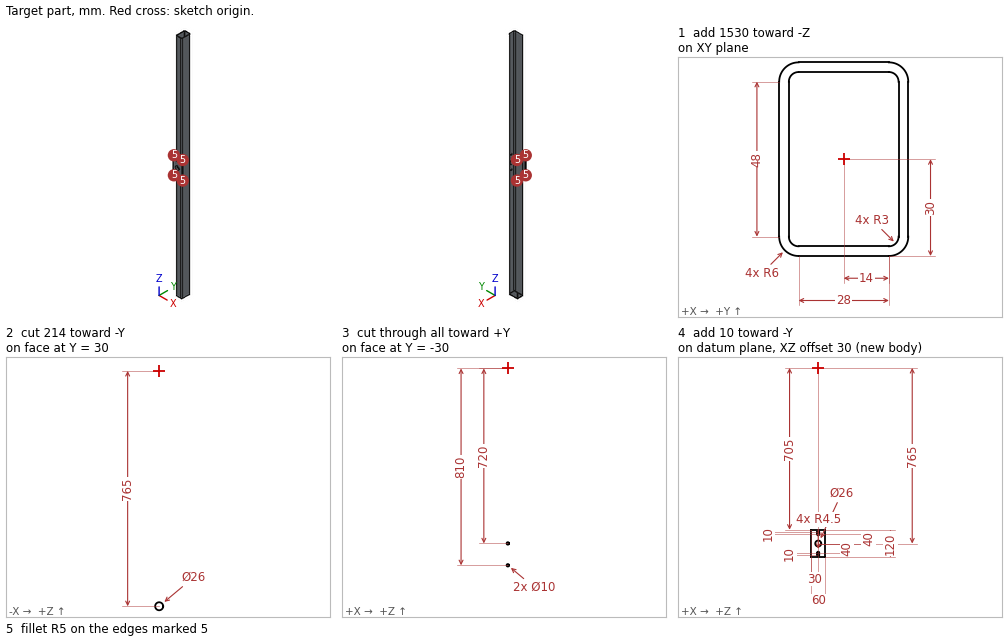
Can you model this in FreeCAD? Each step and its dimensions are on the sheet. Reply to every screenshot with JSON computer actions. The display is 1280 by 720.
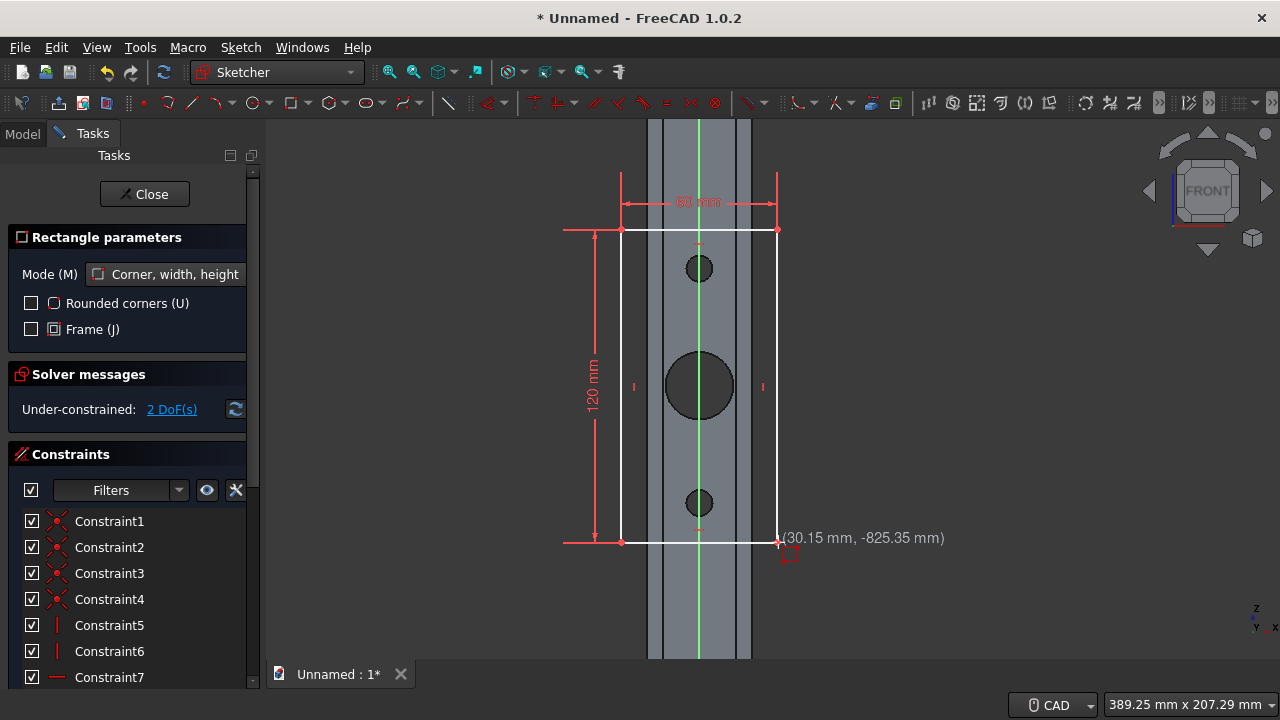
{"action": "left_click", "coordinate": [366, 104]}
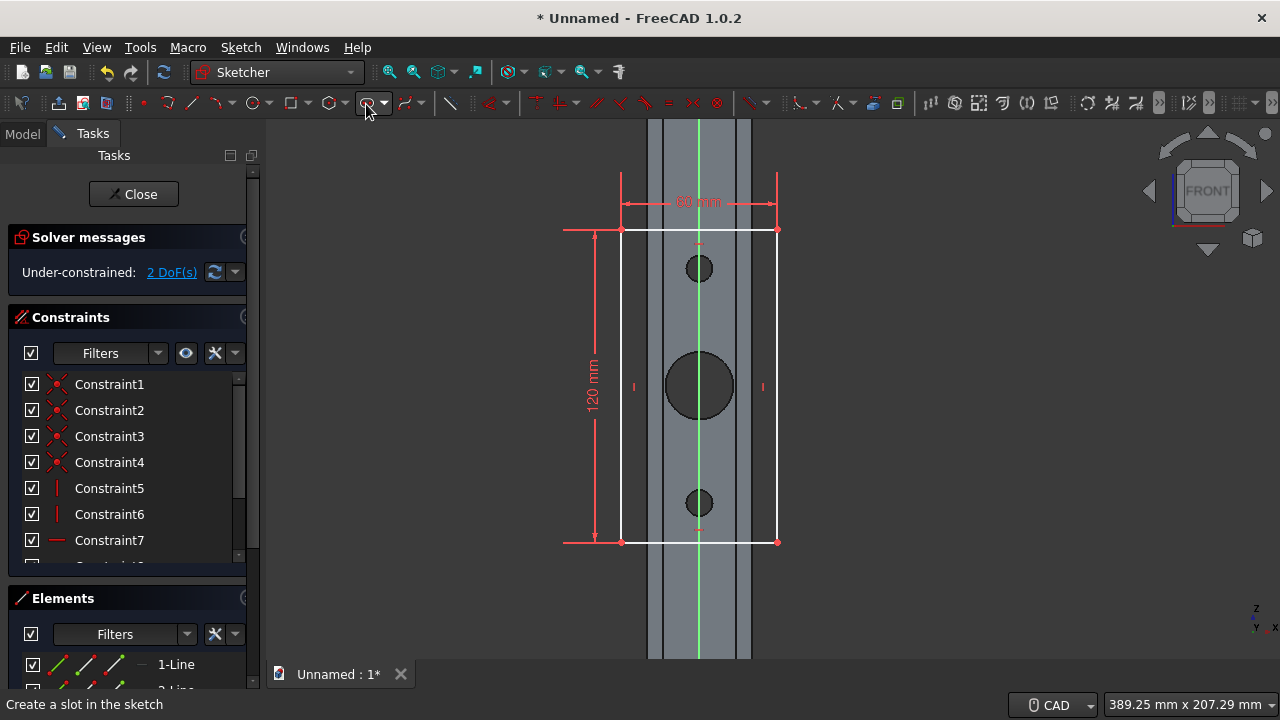
{"action": "scroll", "coordinate": [699, 516], "scroll_direction": "up", "scroll_amount": 4}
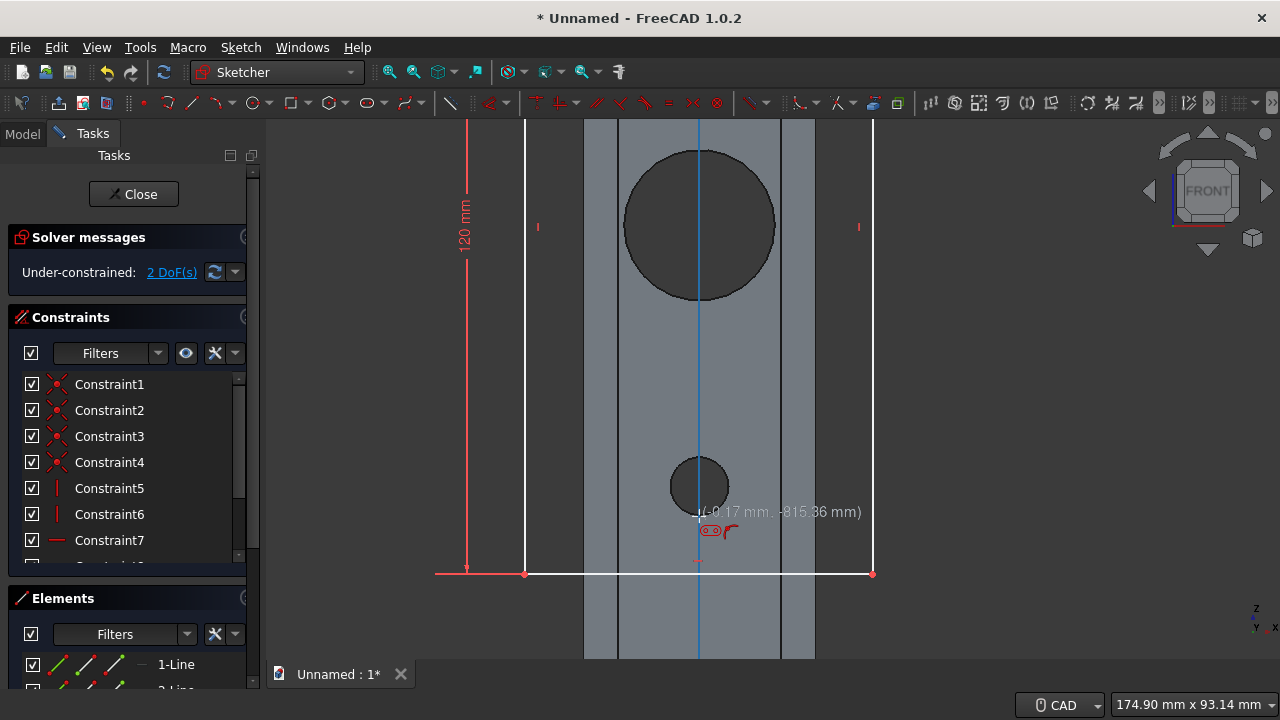
{"action": "left_click", "coordinate": [699, 515]}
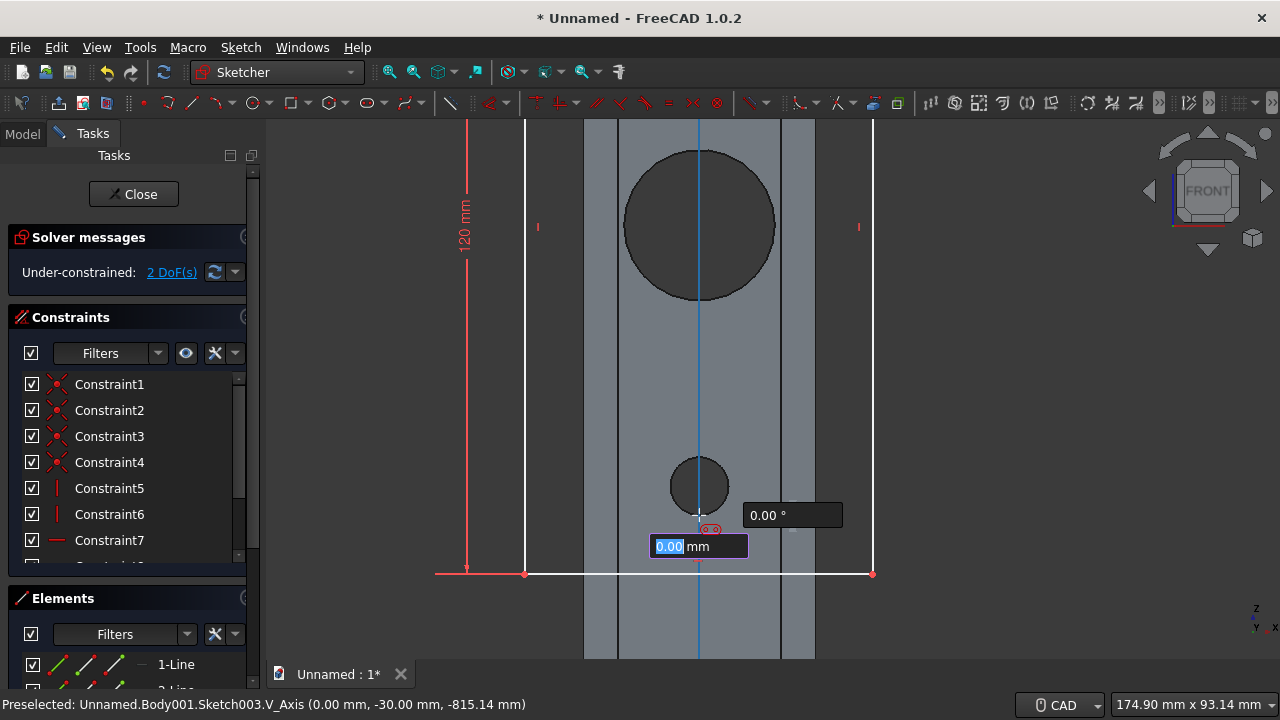
{"action": "left_click", "coordinate": [708, 457]}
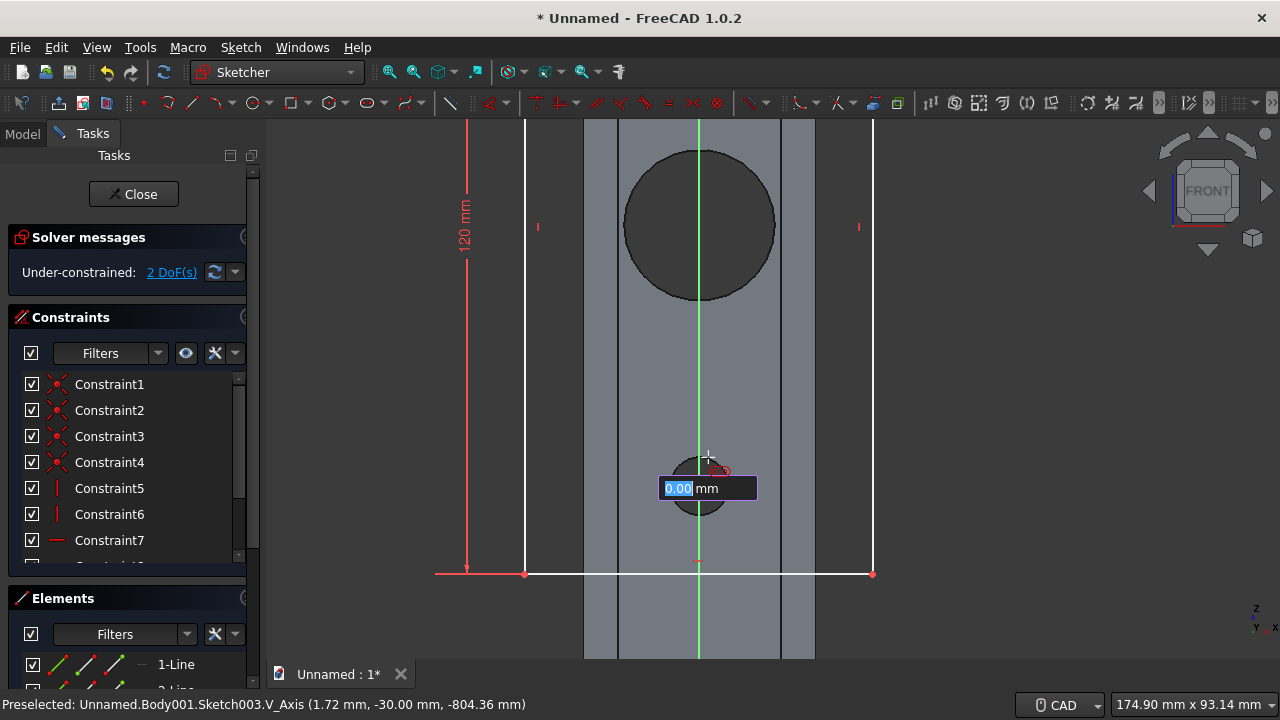
{"action": "left_click", "coordinate": [726, 486]}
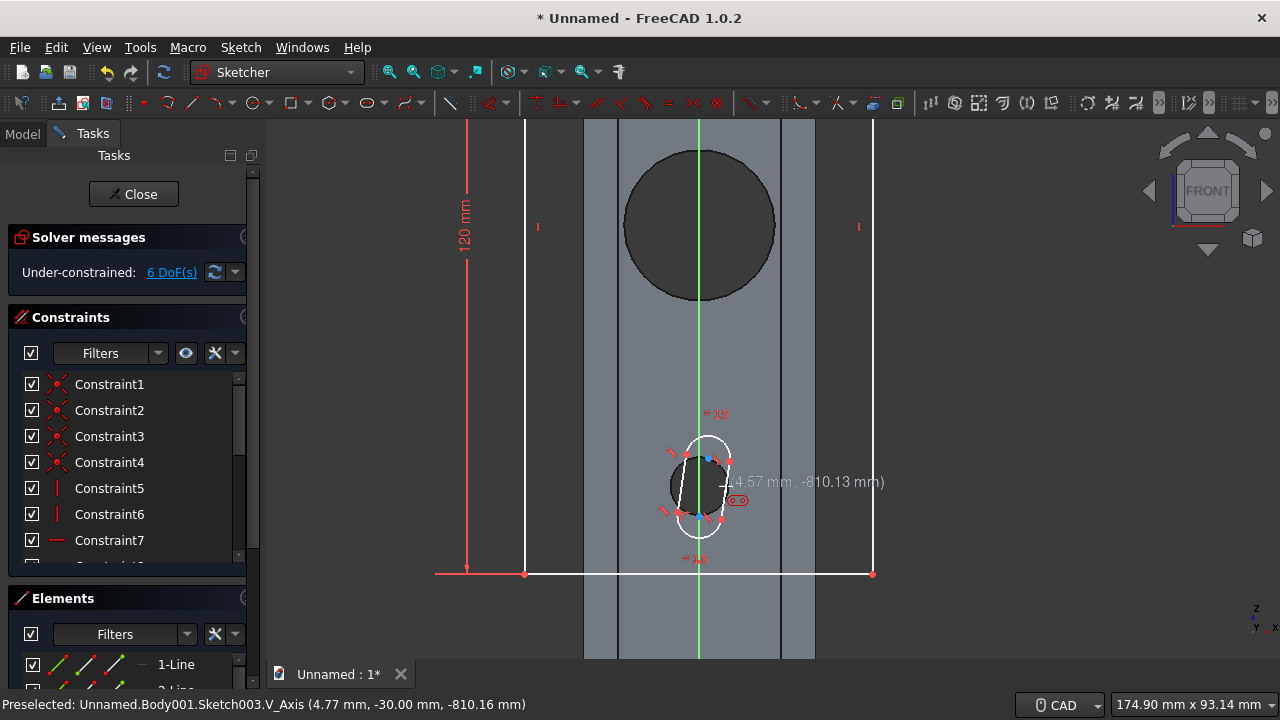
{"action": "scroll", "coordinate": [709, 523], "scroll_direction": "down", "scroll_amount": 4}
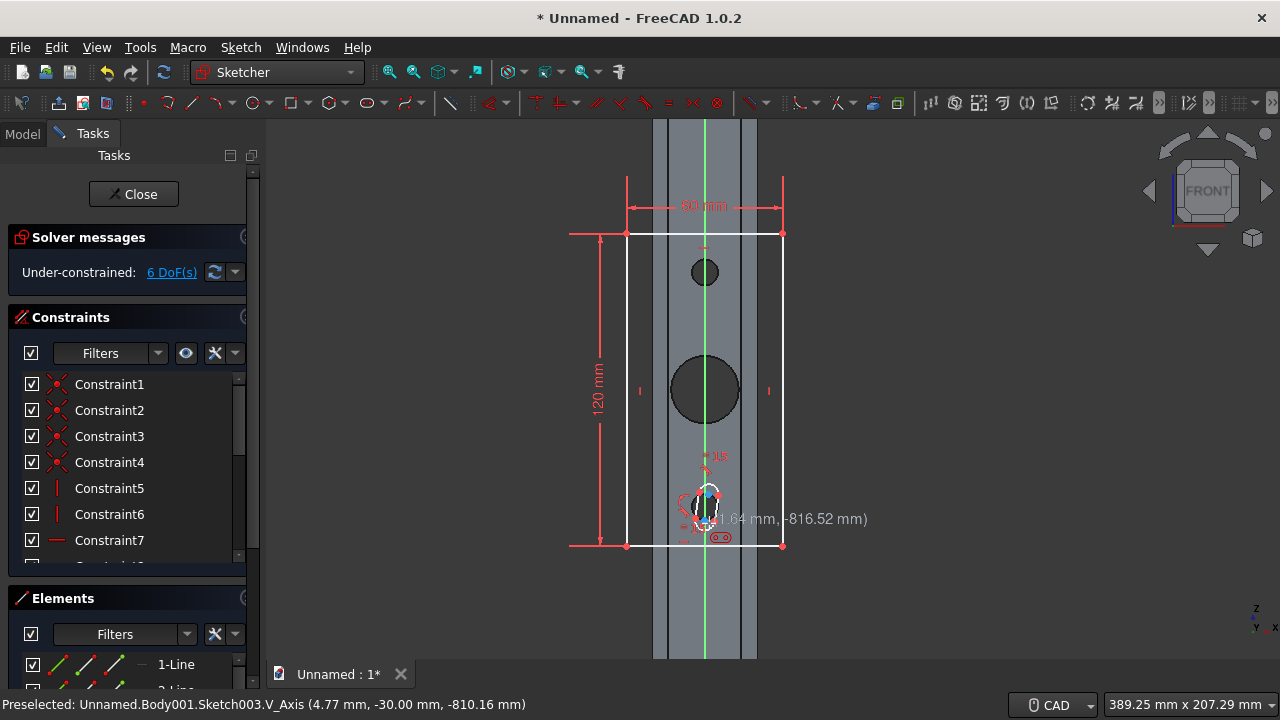
{"action": "scroll", "coordinate": [705, 285], "scroll_direction": "up", "scroll_amount": 4}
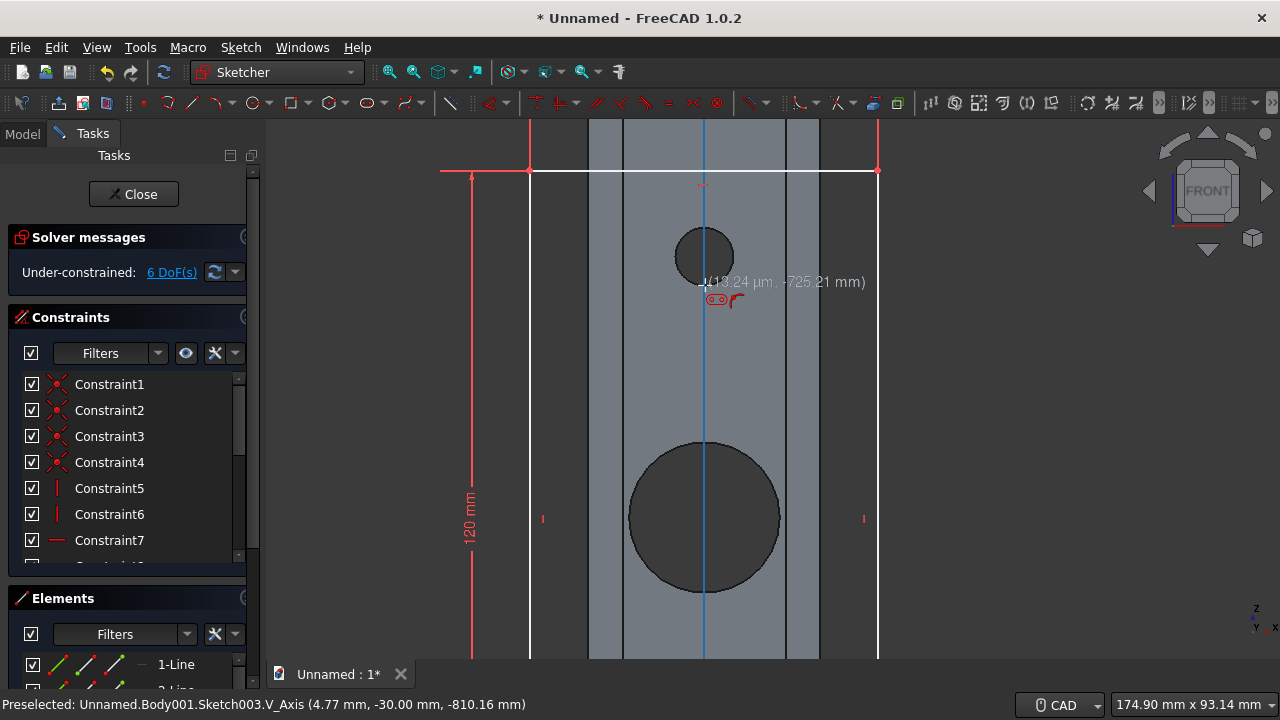
{"action": "left_click", "coordinate": [704, 286]}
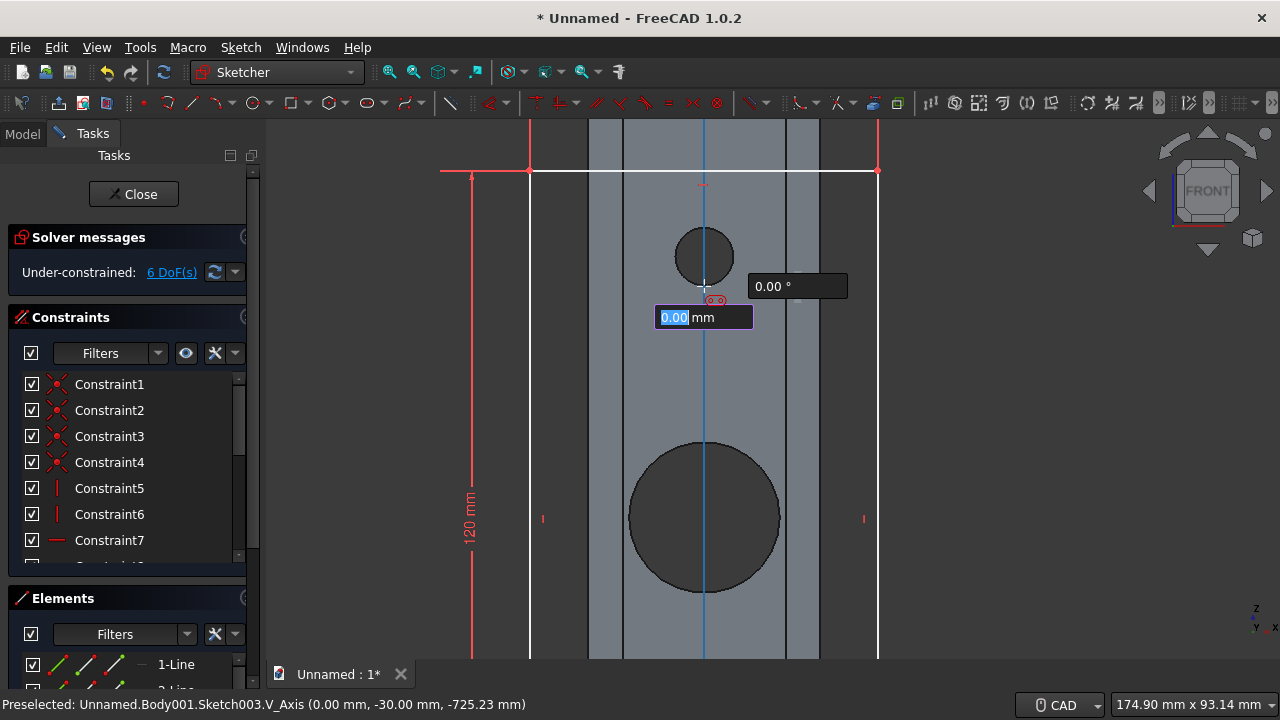
{"action": "left_click", "coordinate": [713, 228]}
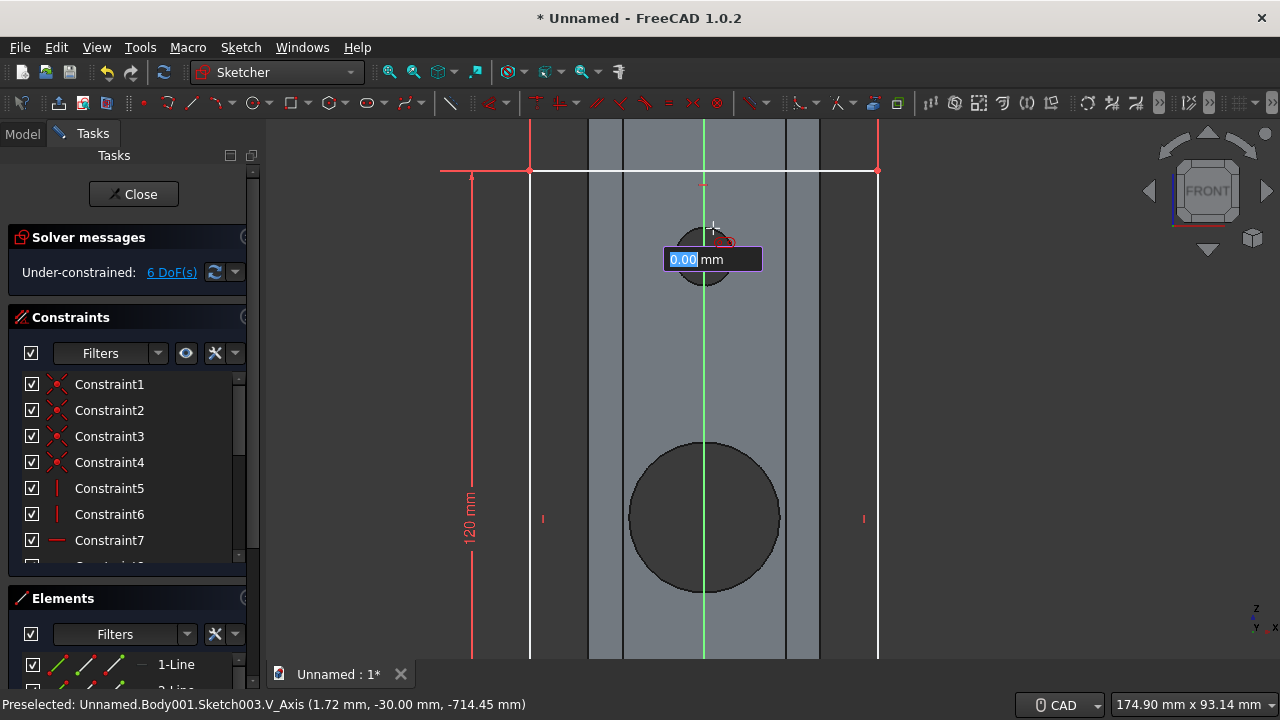
{"action": "left_click", "coordinate": [730, 257]}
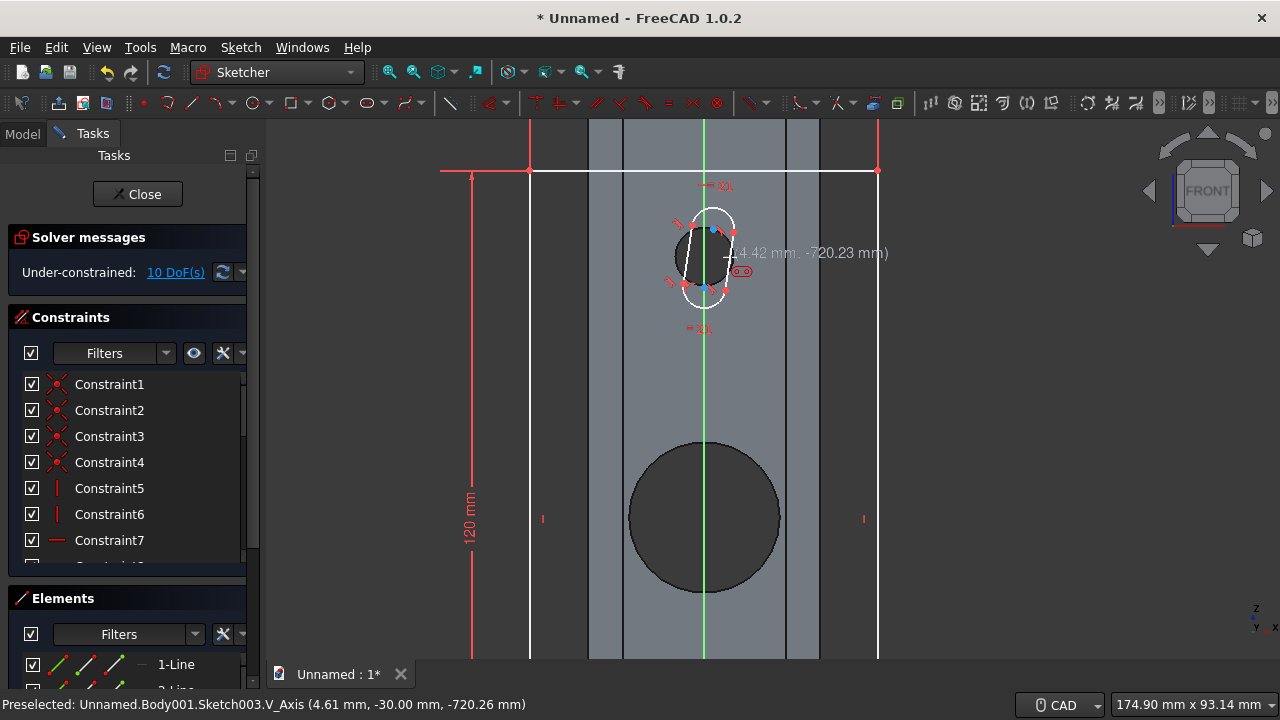
{"action": "left_click", "coordinate": [254, 104]}